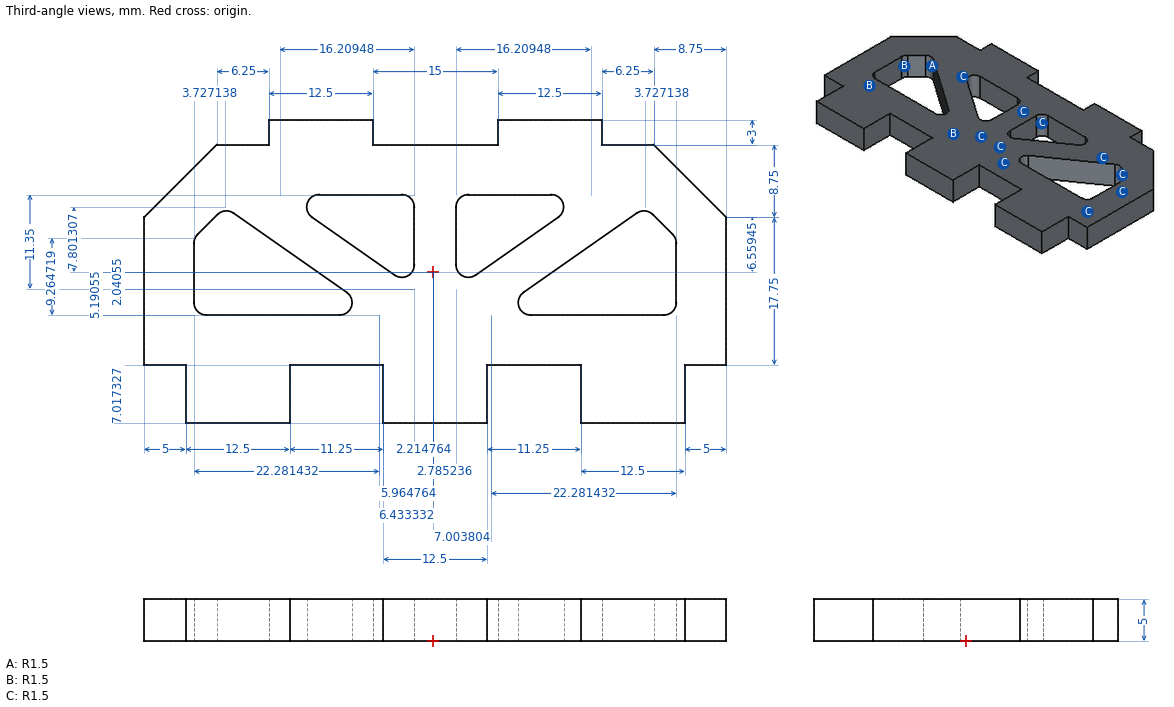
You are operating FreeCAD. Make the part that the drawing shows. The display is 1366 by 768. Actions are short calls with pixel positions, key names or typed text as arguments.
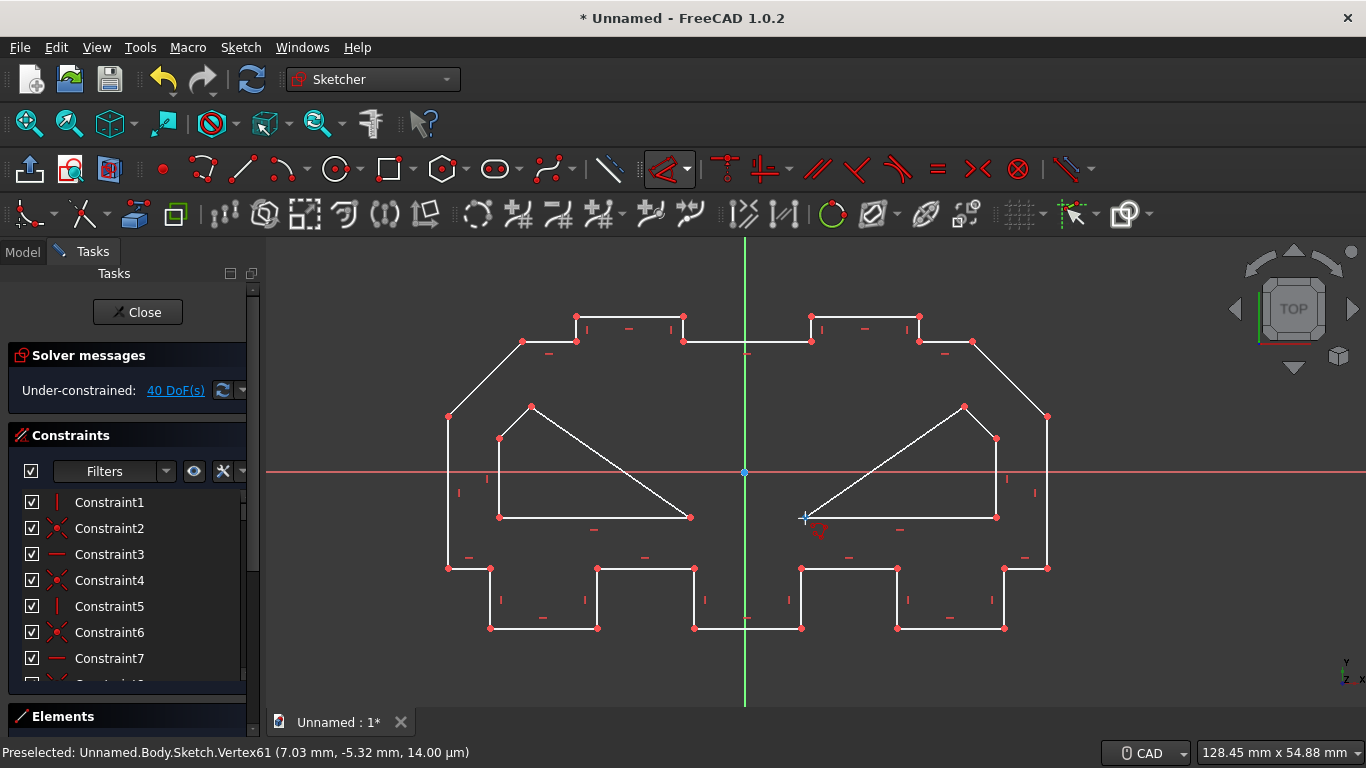
click(726, 490)
click(587, 393)
click(726, 393)
click(726, 491)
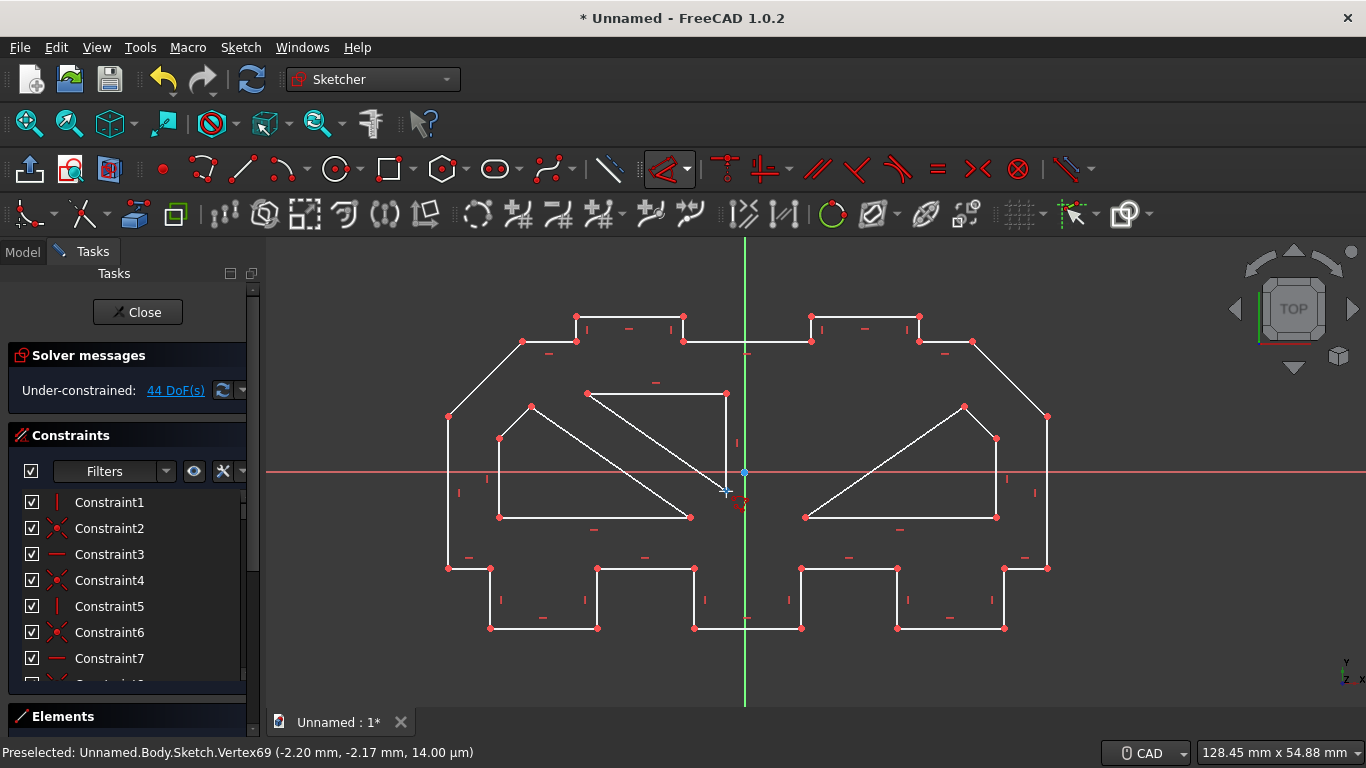
click(769, 490)
click(769, 393)
click(907, 393)
click(769, 491)
key(Escape)
key(Escape)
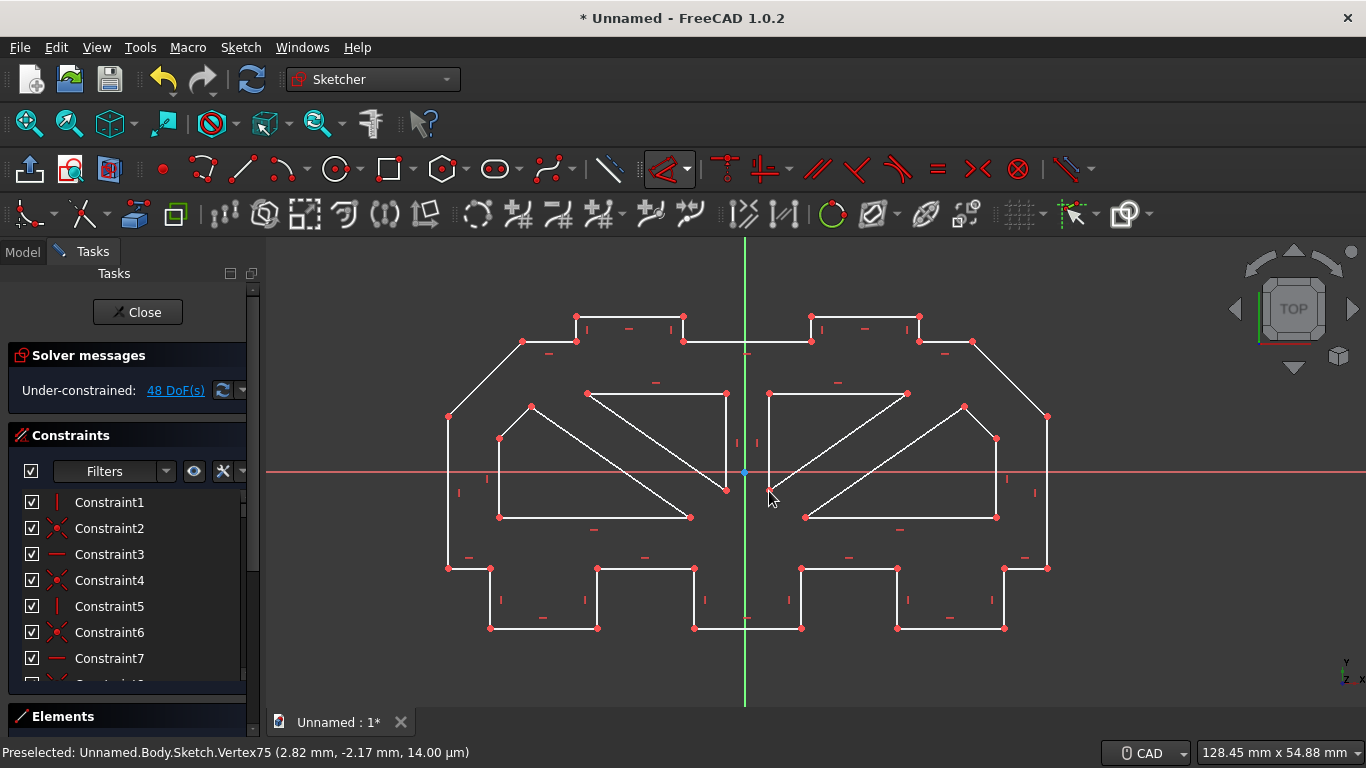
key(d)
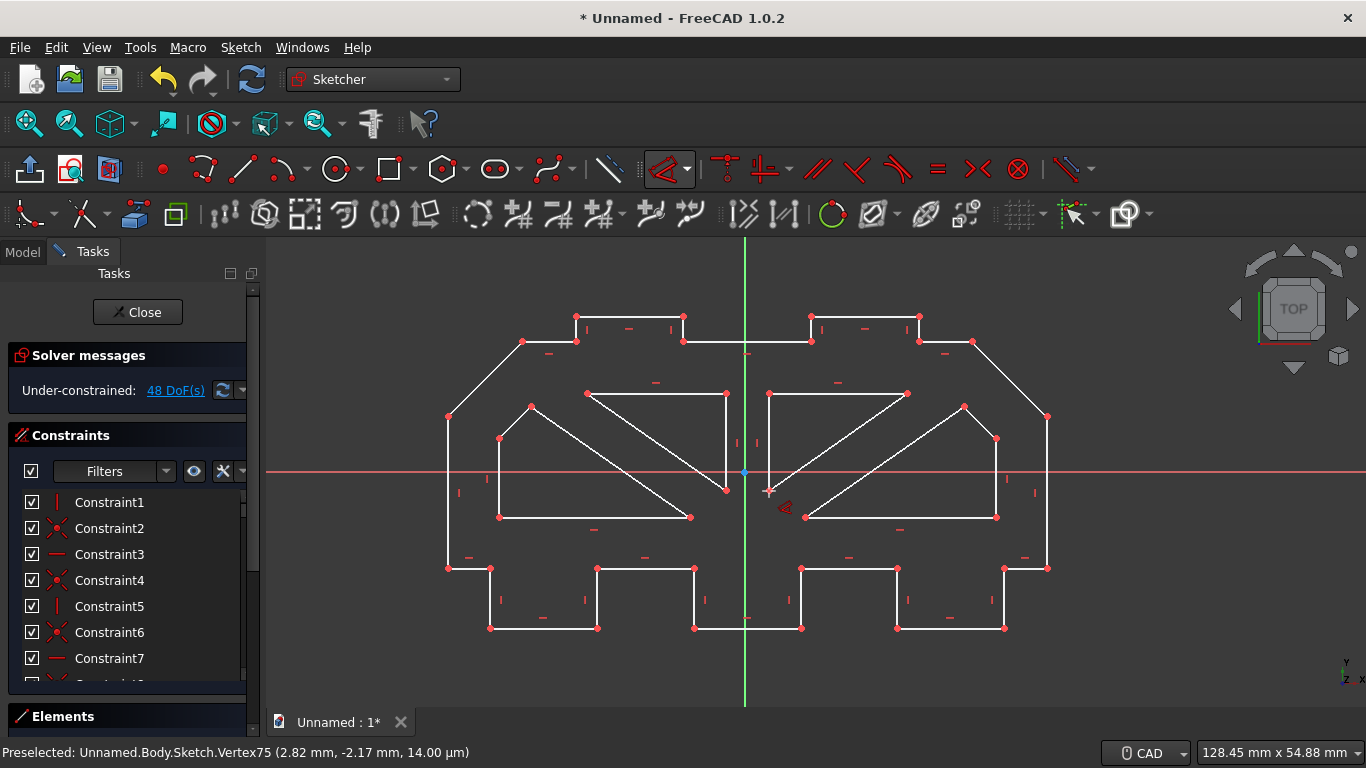
click(1017, 569)
click(1025, 603)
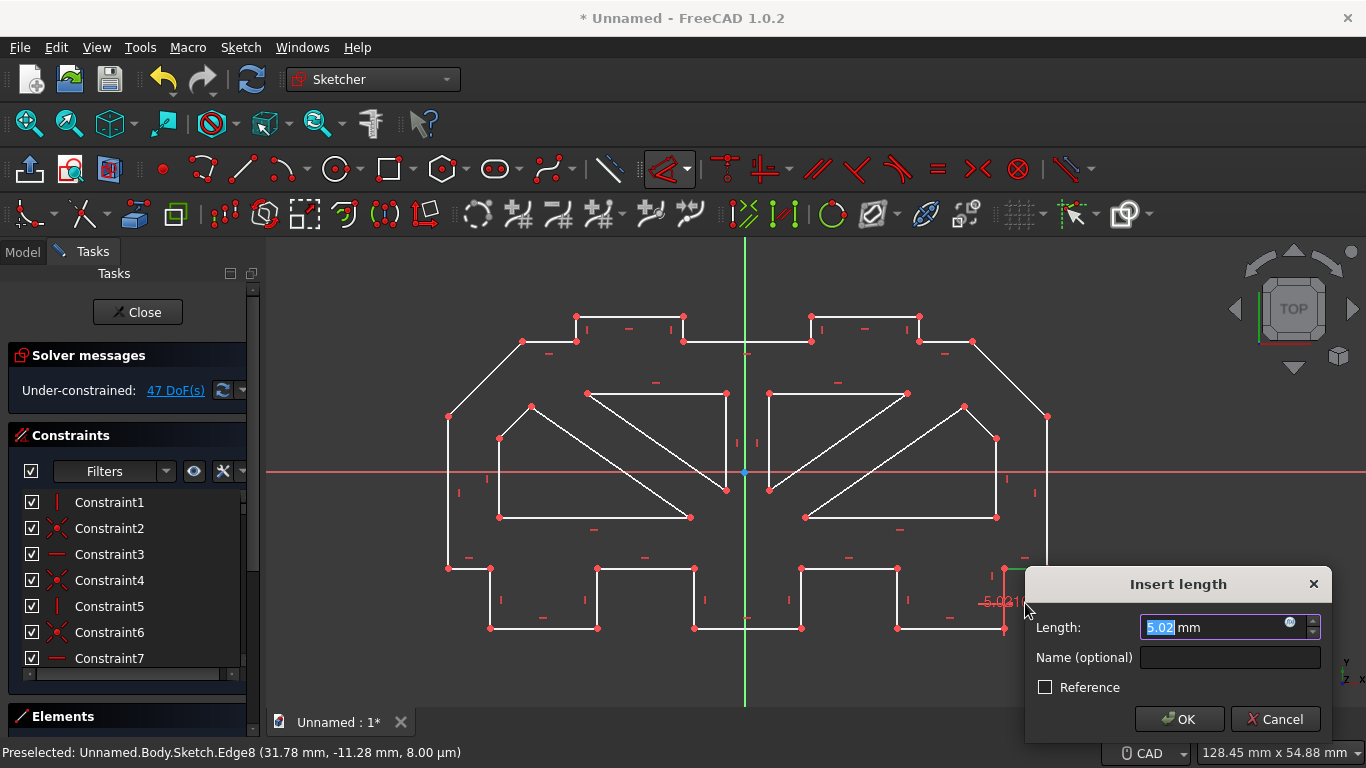
text(5)
key(Return)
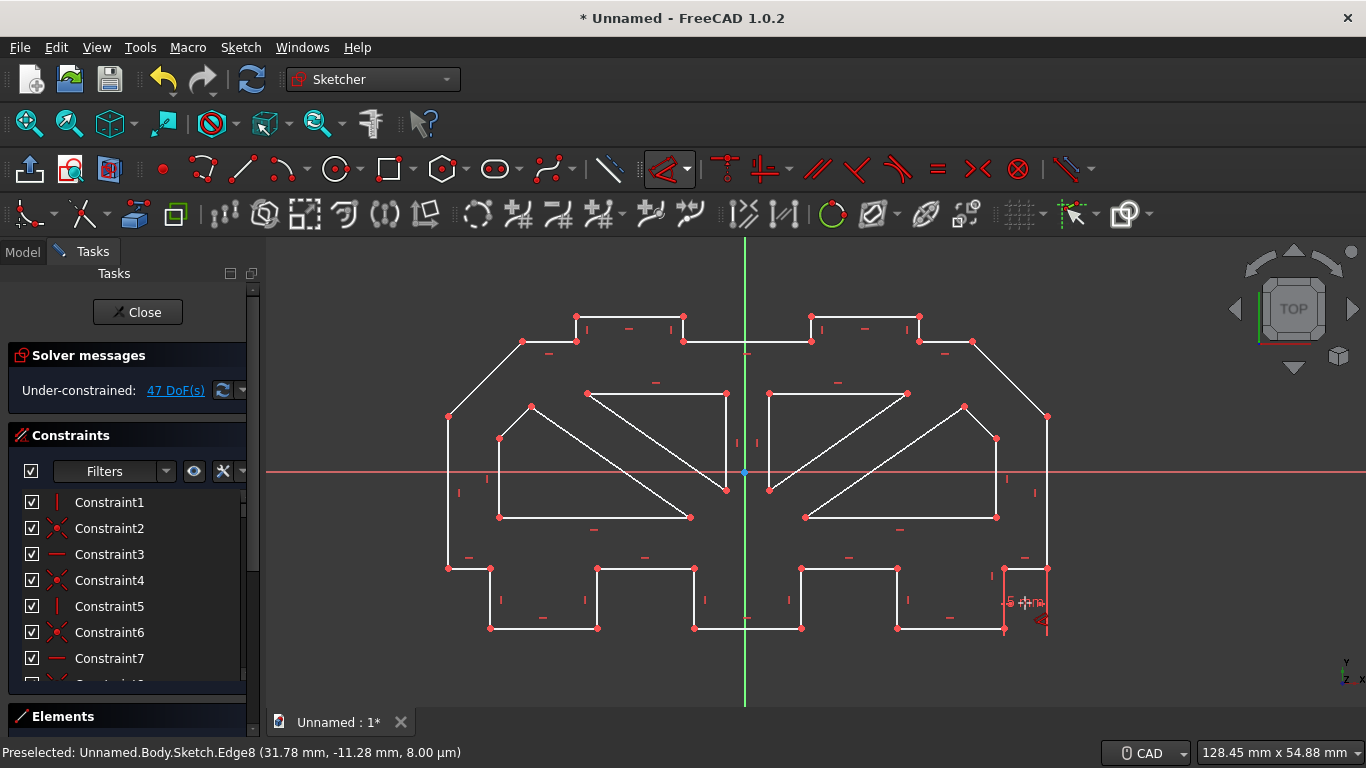
scroll(919, 332, up, 3)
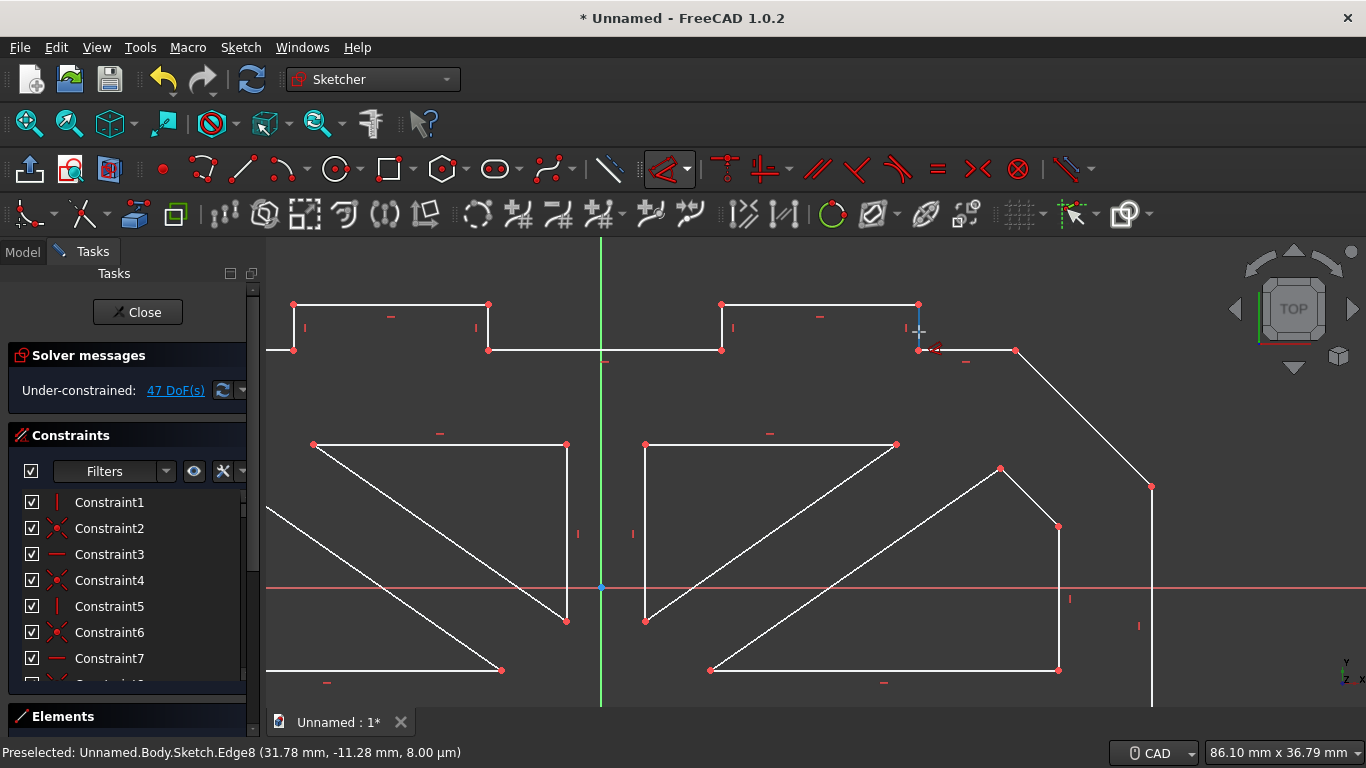
click(919, 332)
click(953, 327)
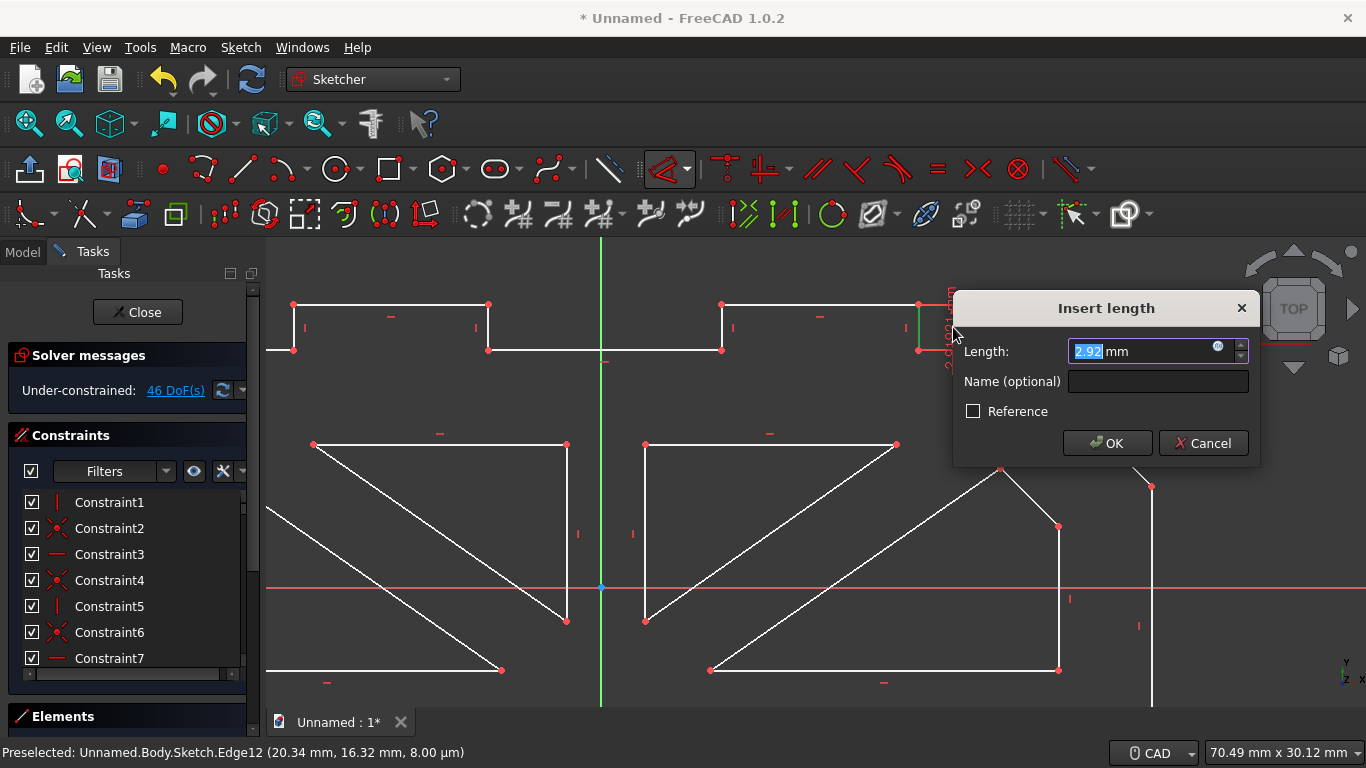
text(3)
key(Return)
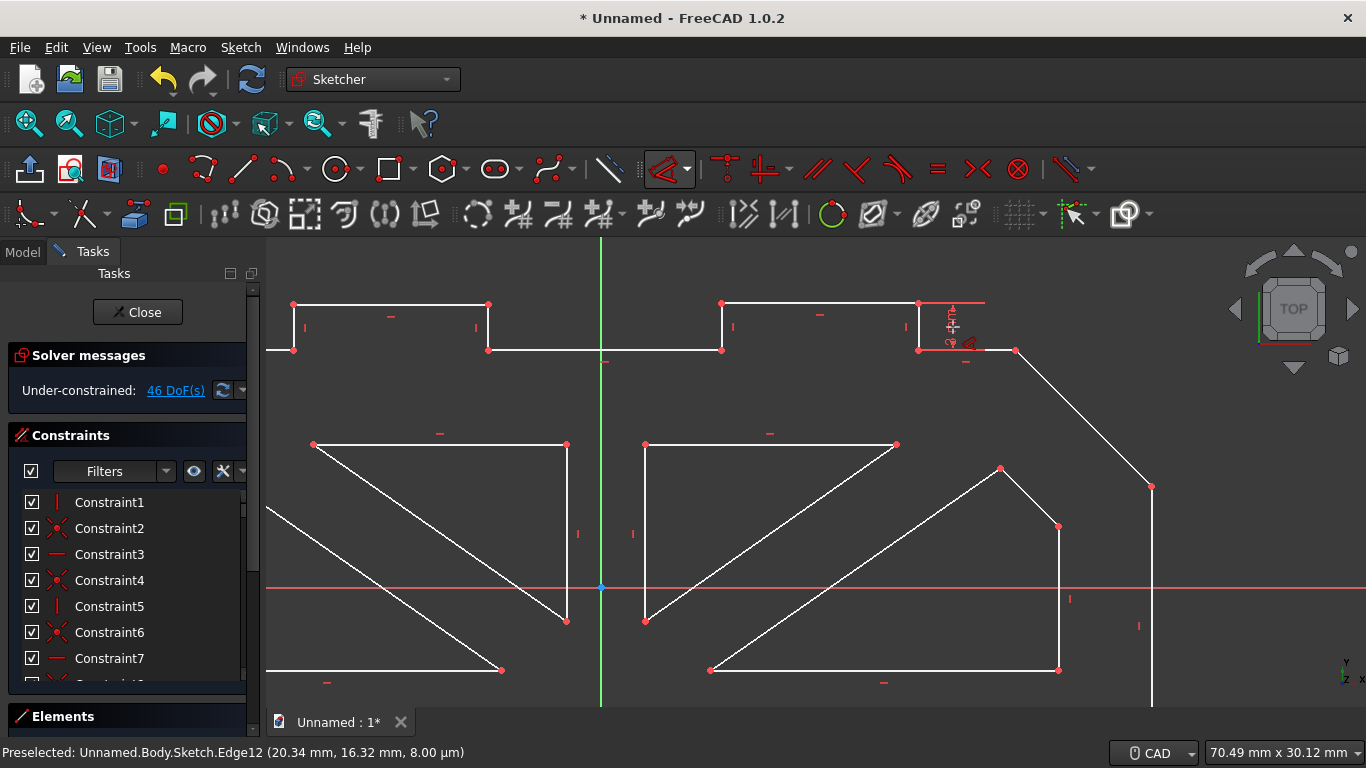
click(722, 317)
click(756, 327)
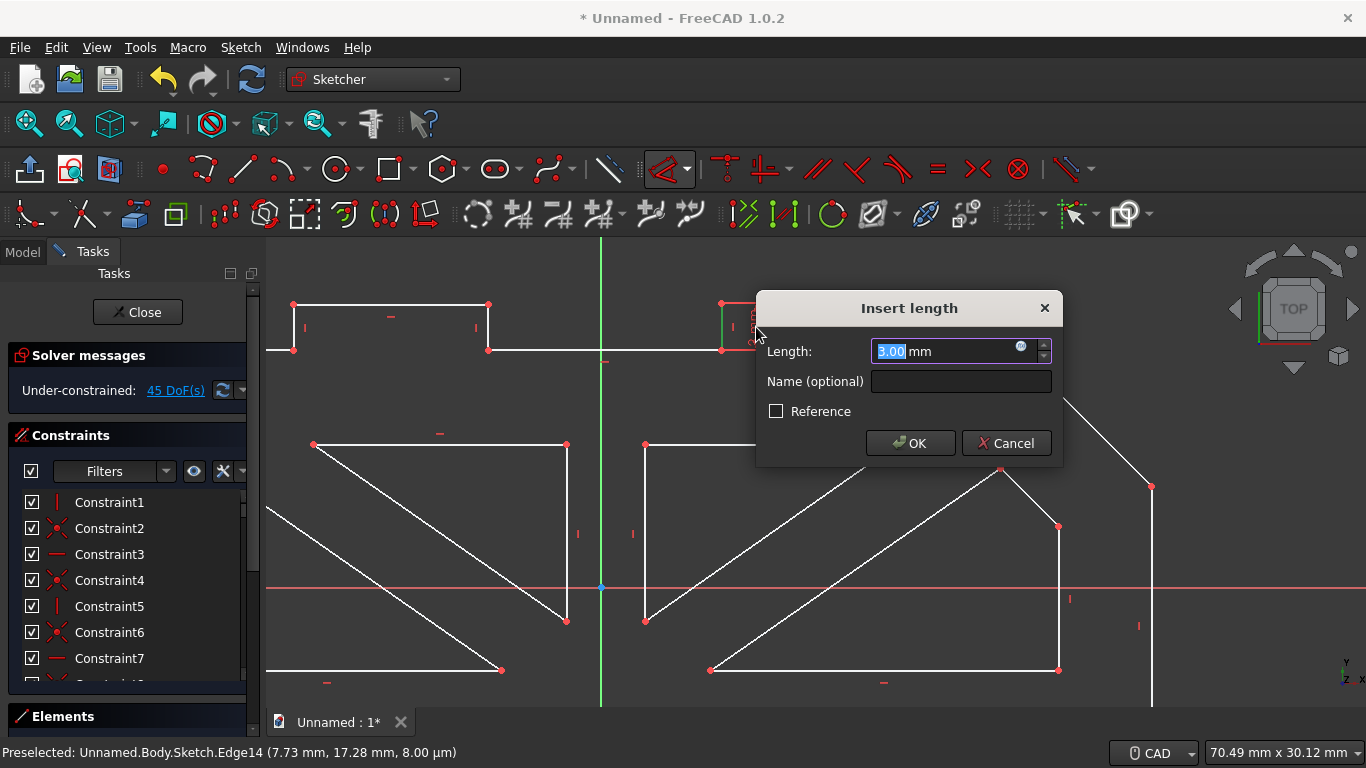
text(3)
key(Return)